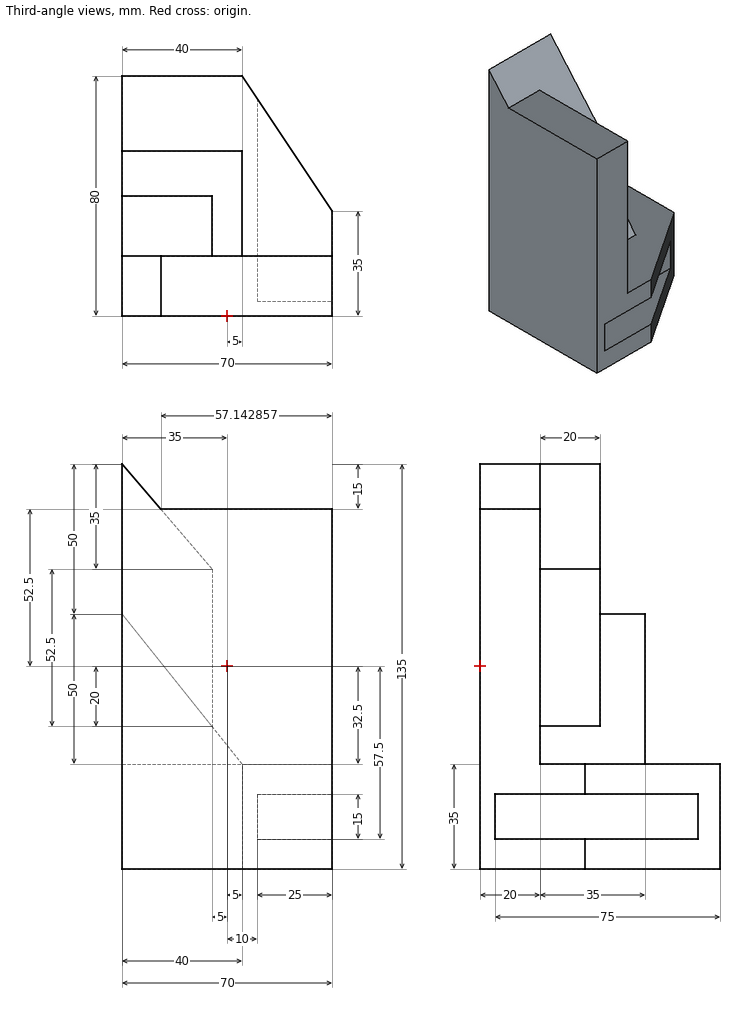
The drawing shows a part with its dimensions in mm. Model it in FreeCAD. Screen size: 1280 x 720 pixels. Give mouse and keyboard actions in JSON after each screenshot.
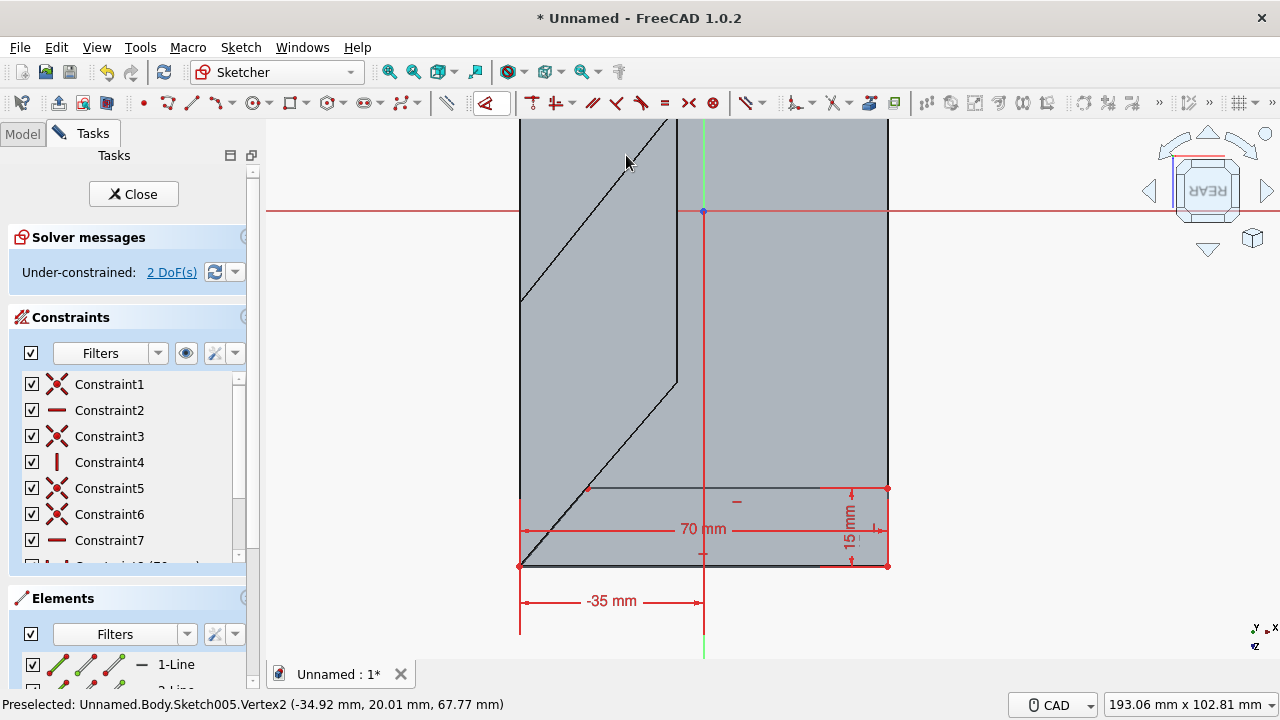
{"action": "left_click", "coordinate": [587, 488]}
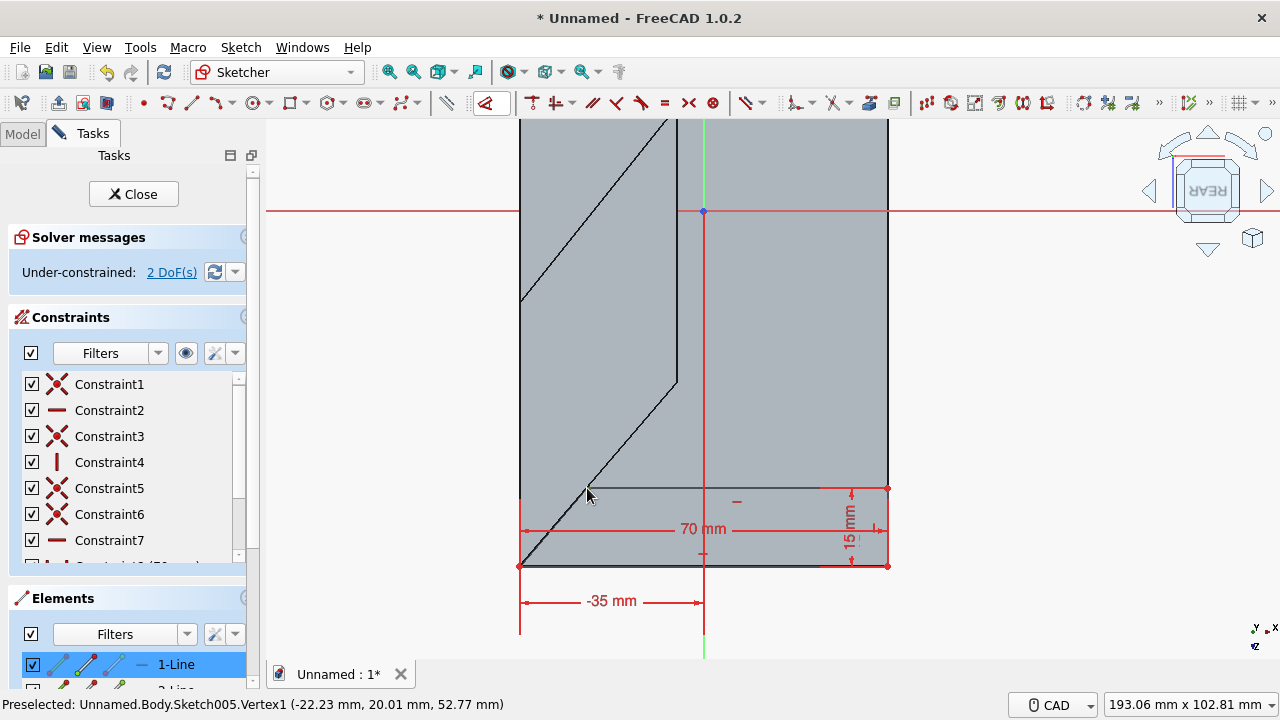
{"action": "key", "text": "i"}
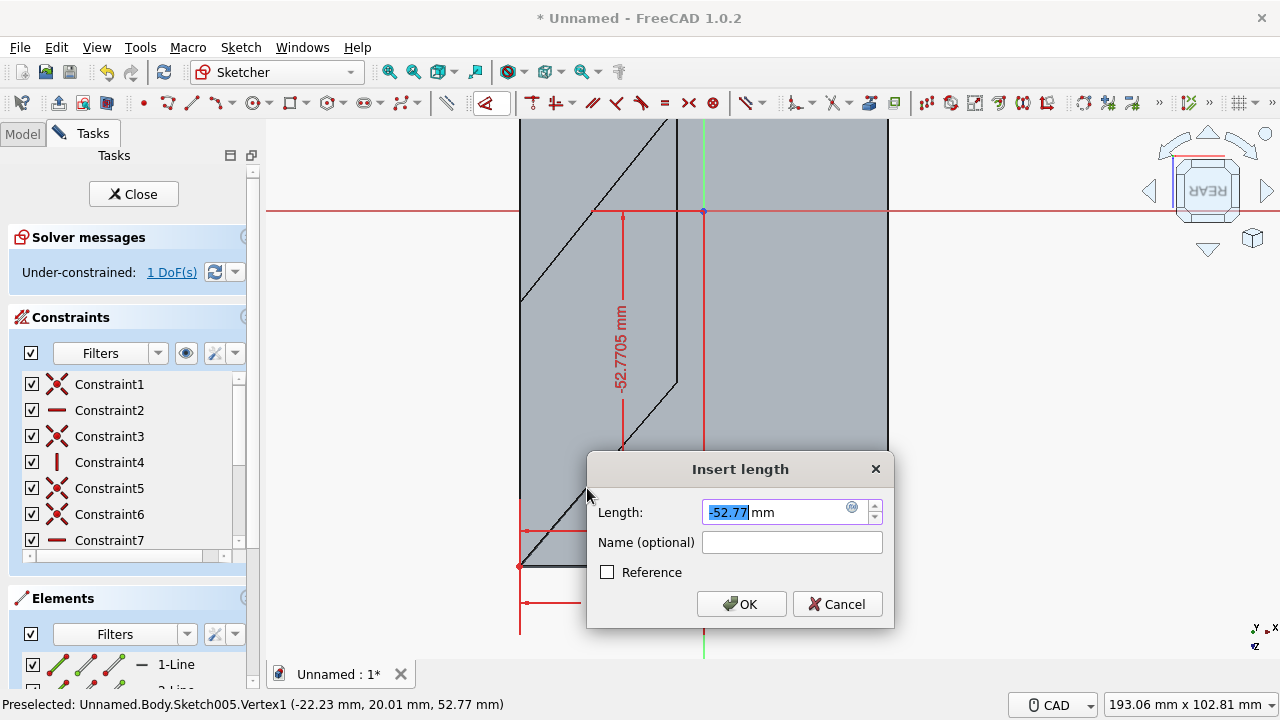
{"action": "type", "text": "-52.5"}
{"action": "key", "text": "Return"}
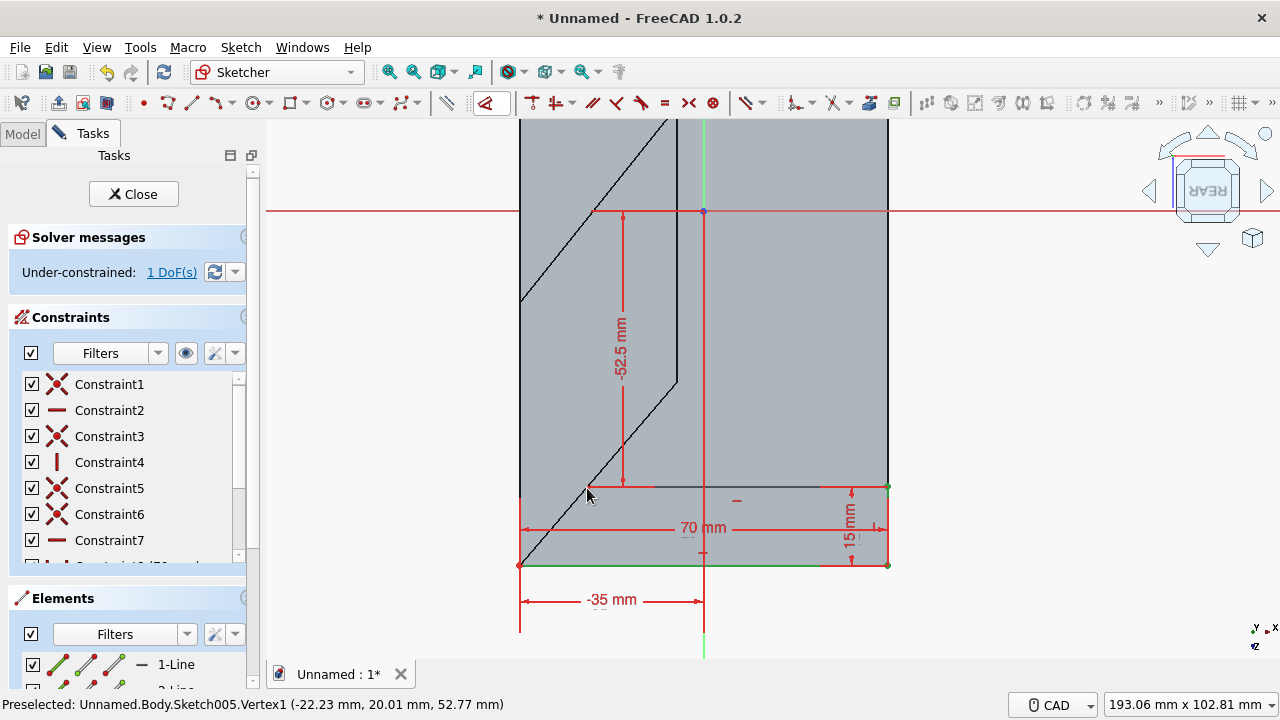
{"action": "left_click", "coordinate": [797, 487]}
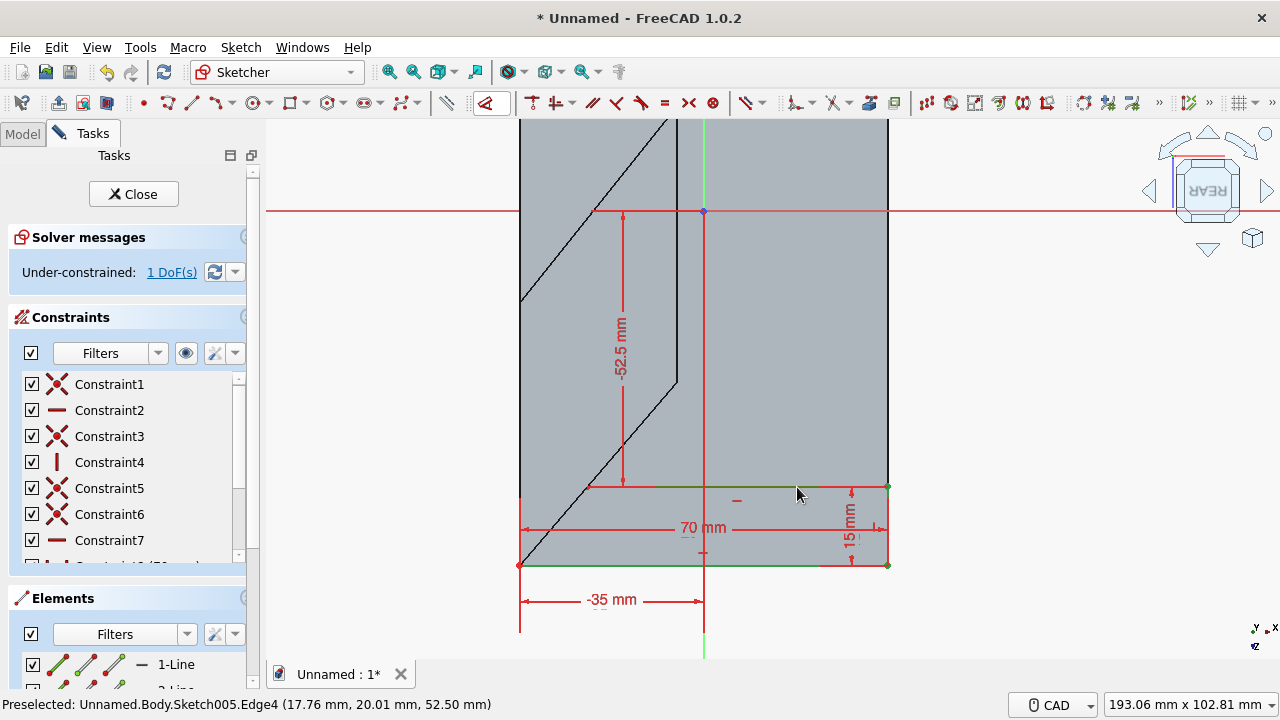
{"action": "left_click", "coordinate": [504, 104]}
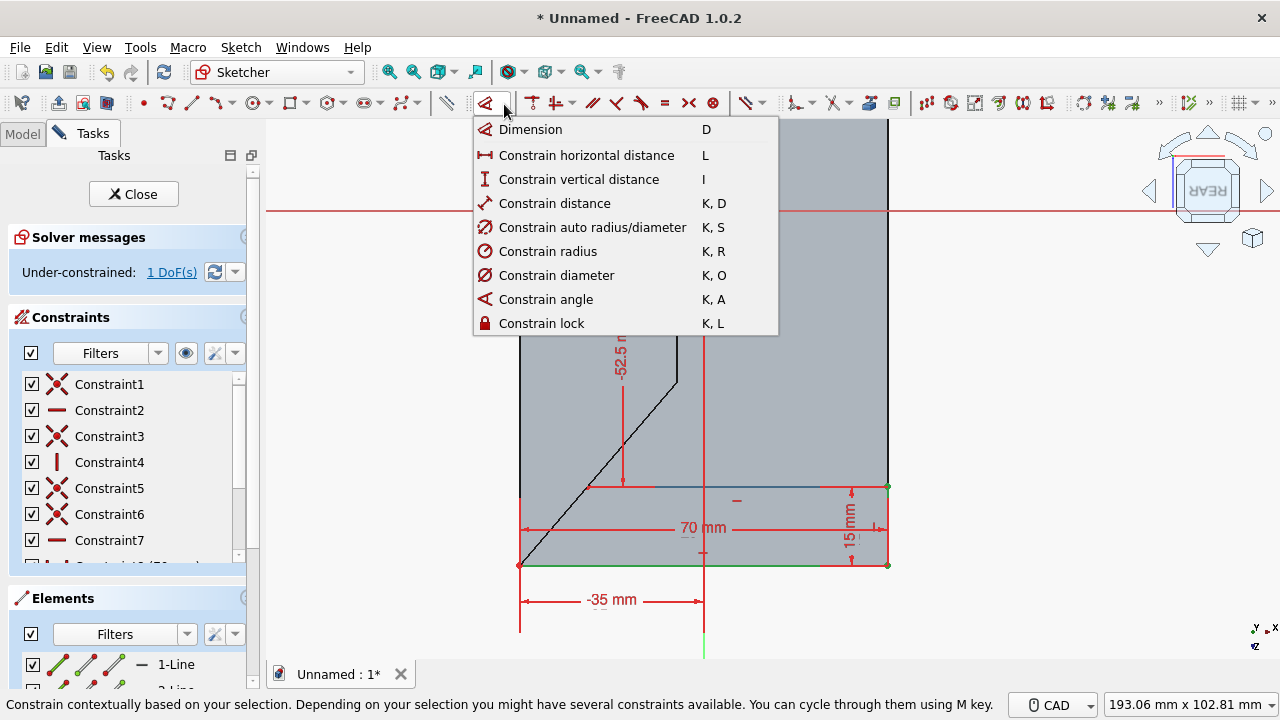
{"action": "left_click", "coordinate": [626, 155]}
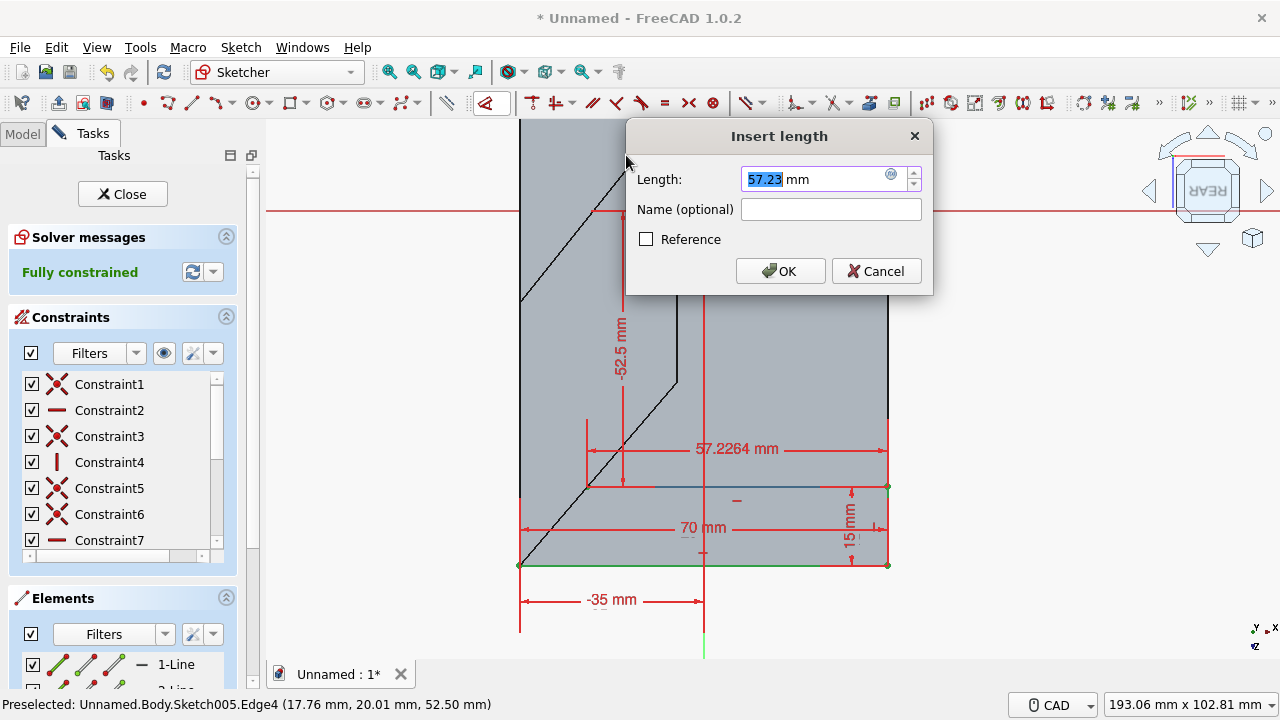
{"action": "type", "text": "57.142857"}
{"action": "key", "text": "Return"}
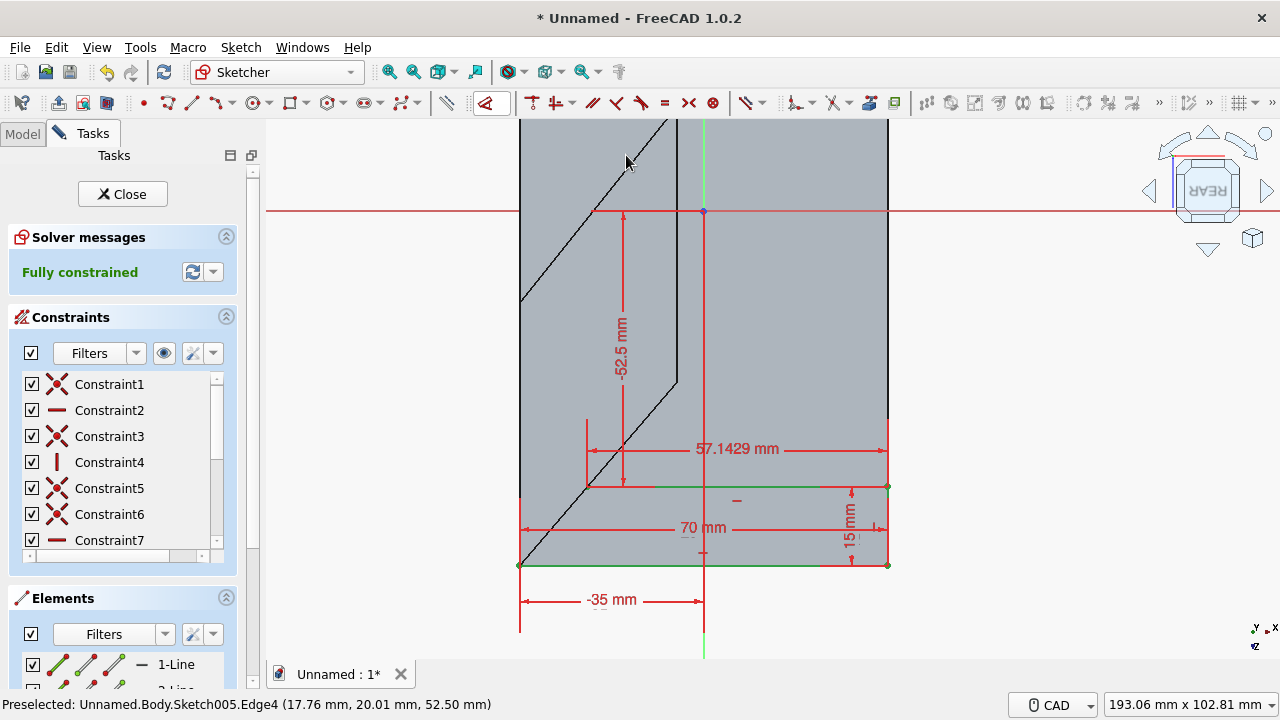
{"action": "left_click", "coordinate": [123, 194]}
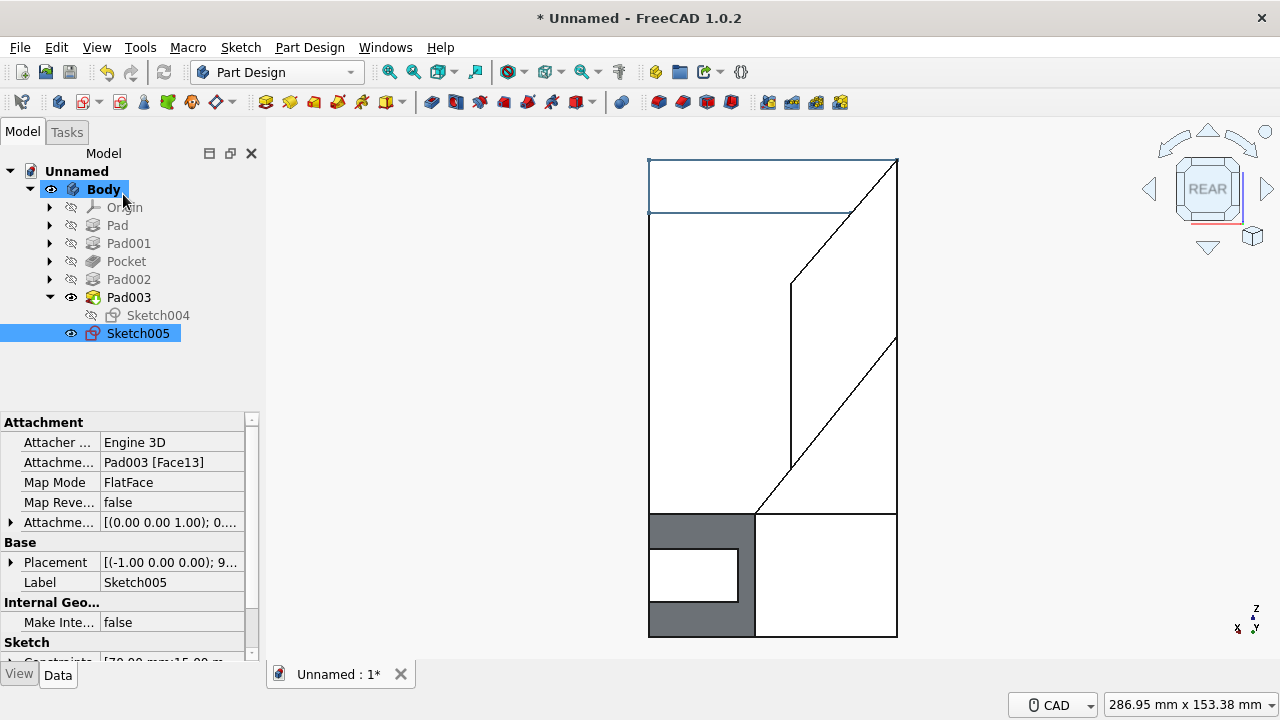
{"action": "left_click", "coordinate": [432, 102]}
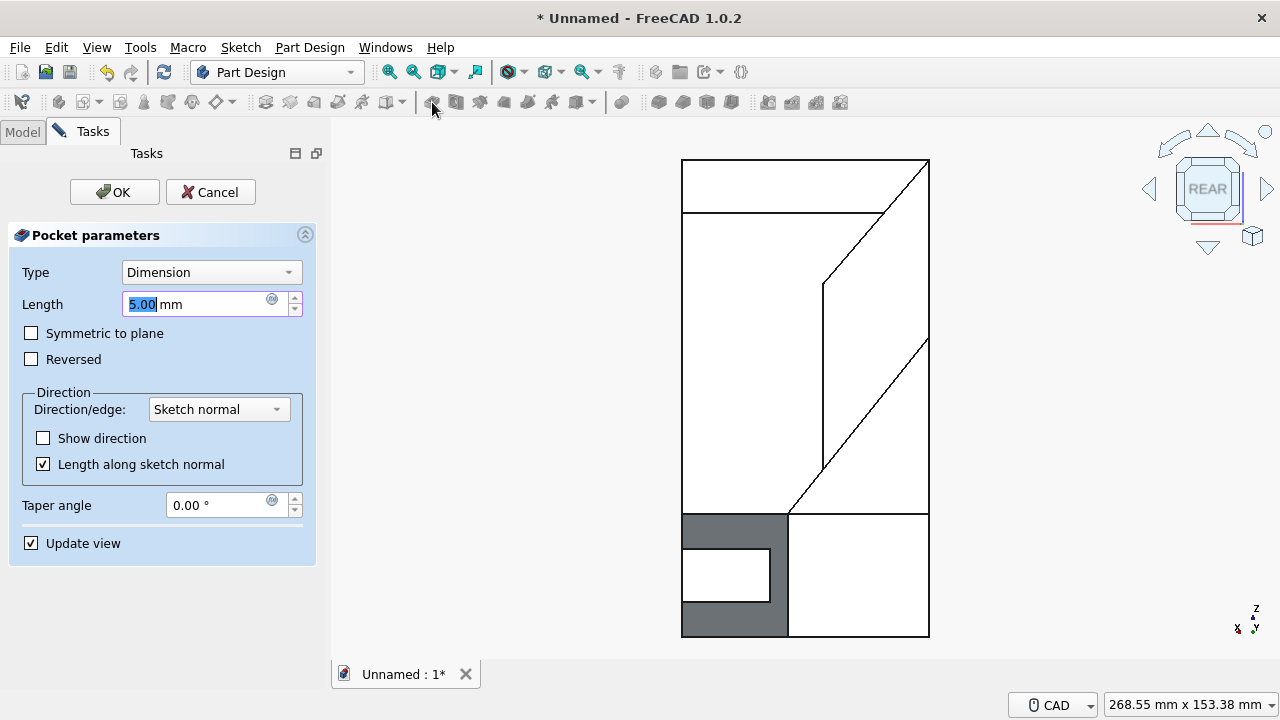
{"action": "type", "text": "20"}
{"action": "key", "text": "Tab"}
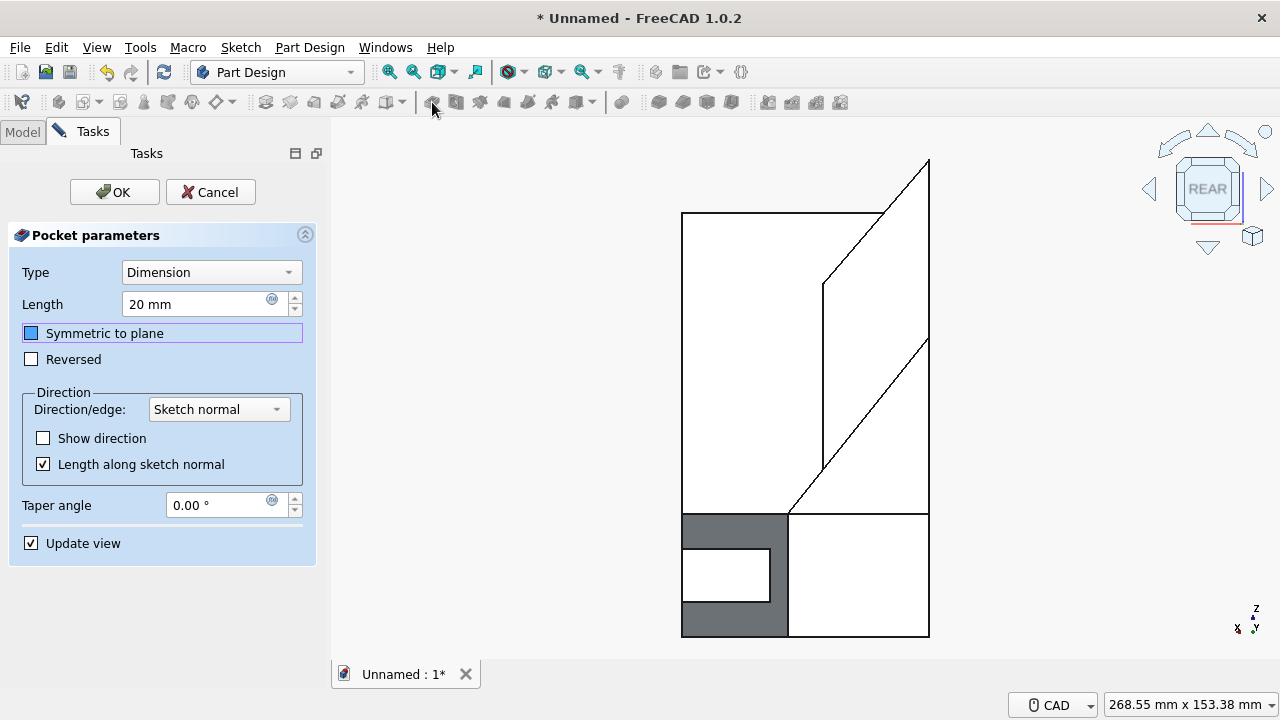
{"action": "left_click", "coordinate": [115, 192]}